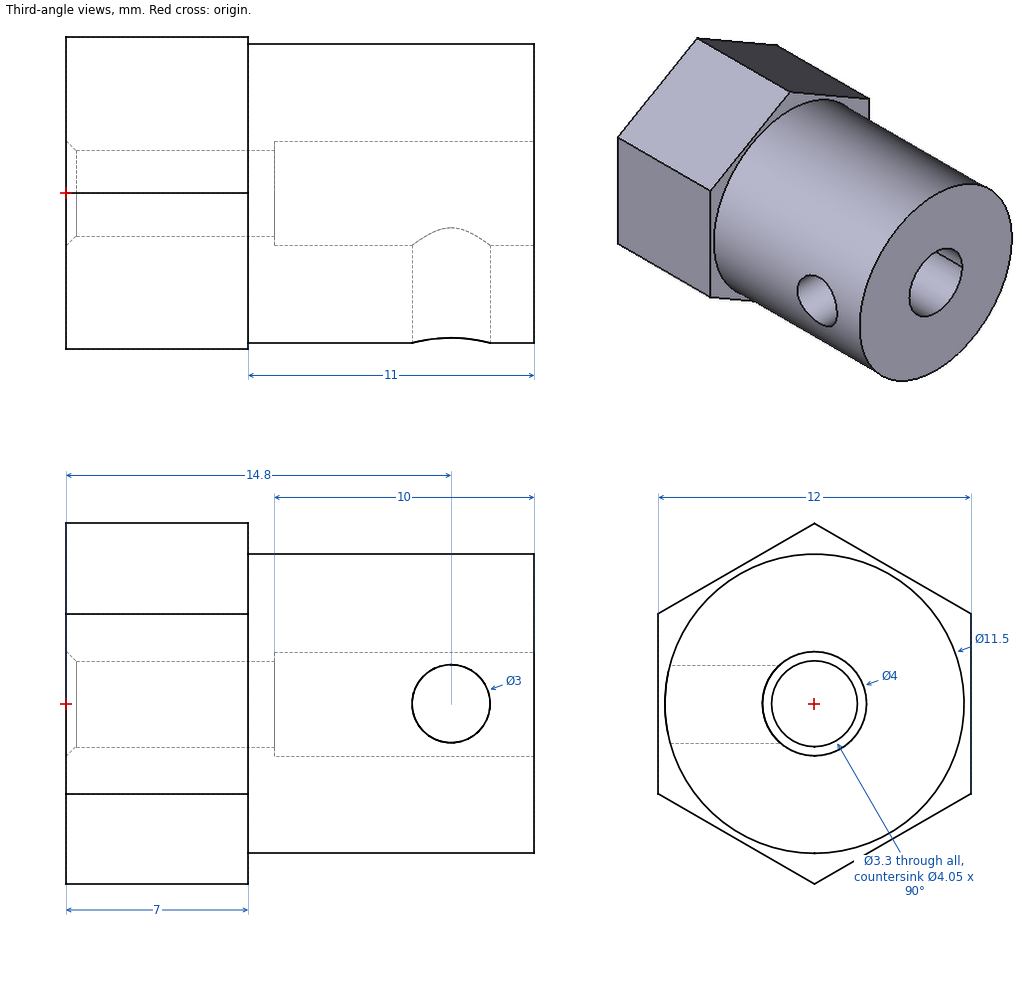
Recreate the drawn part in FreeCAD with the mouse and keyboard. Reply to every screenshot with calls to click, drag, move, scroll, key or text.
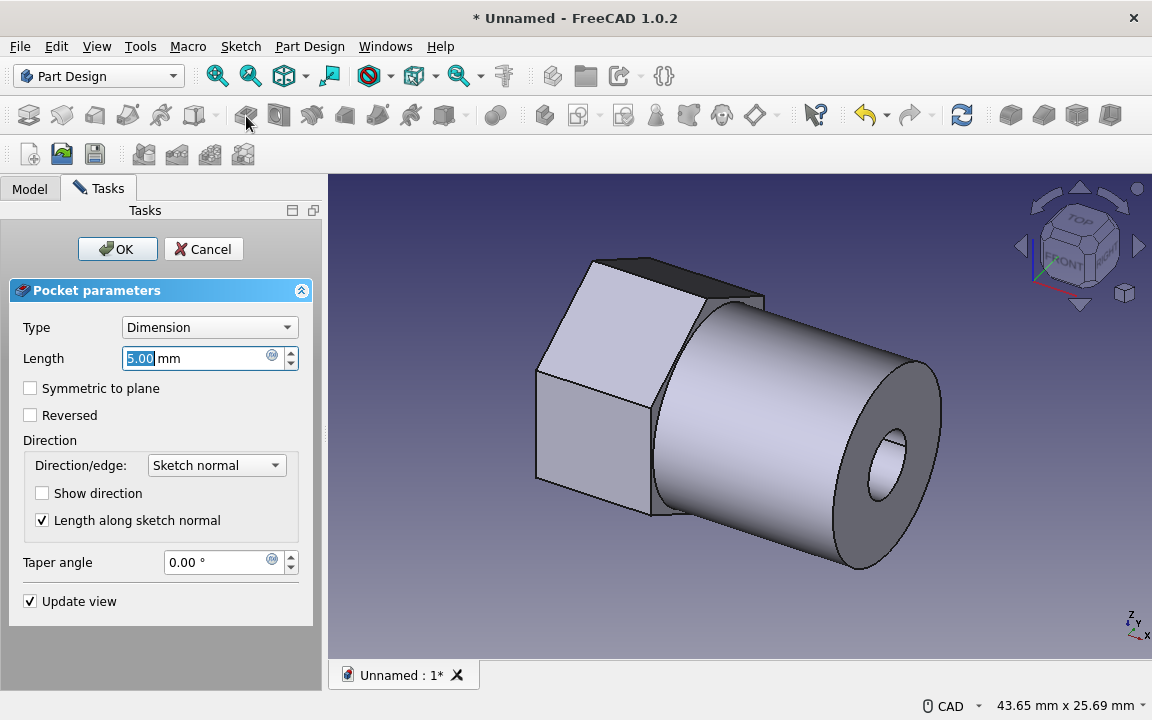
click(210, 328)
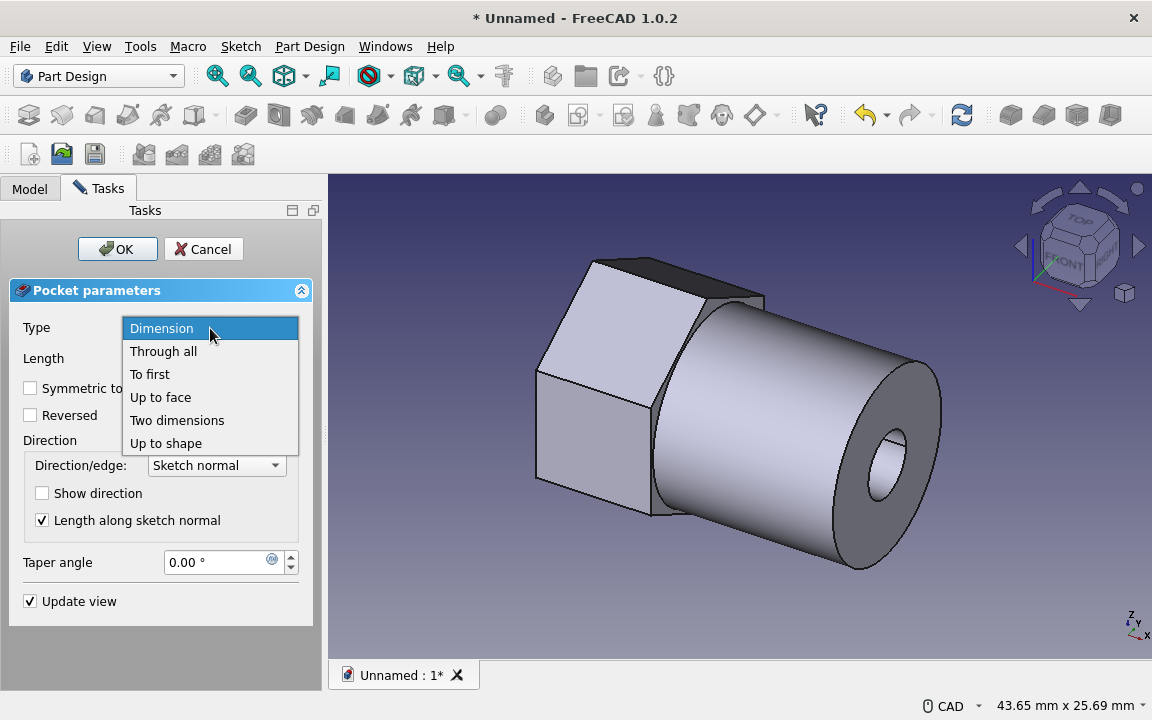
click(208, 352)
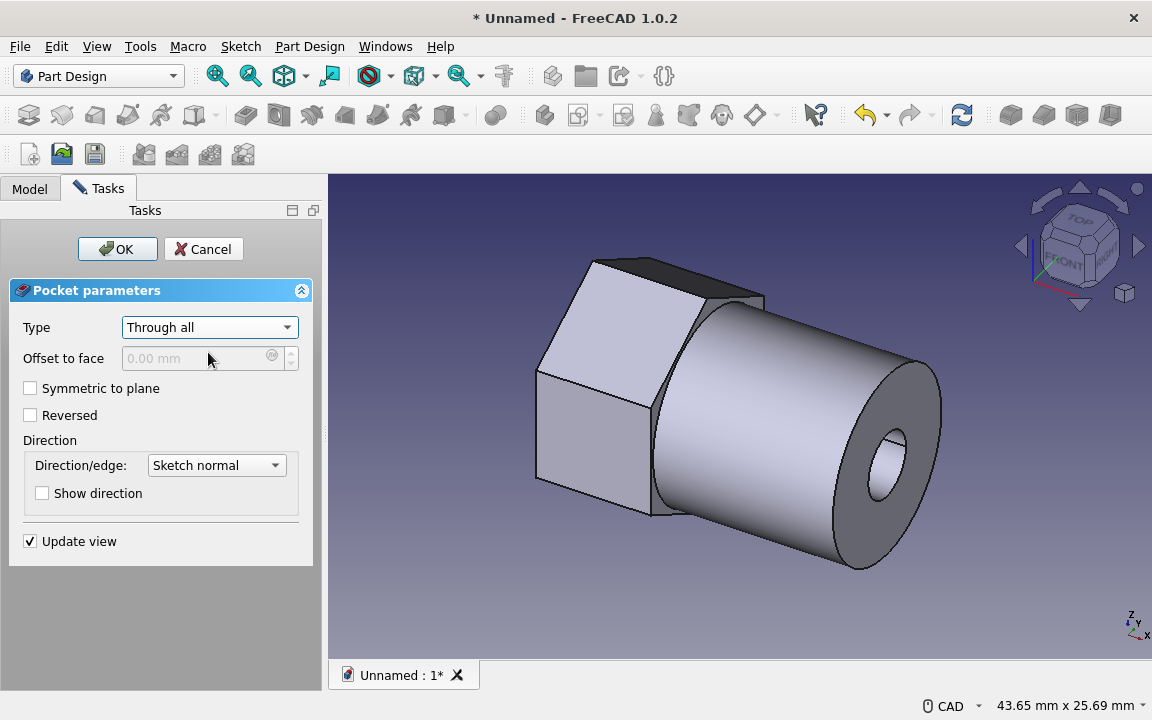
click(31, 415)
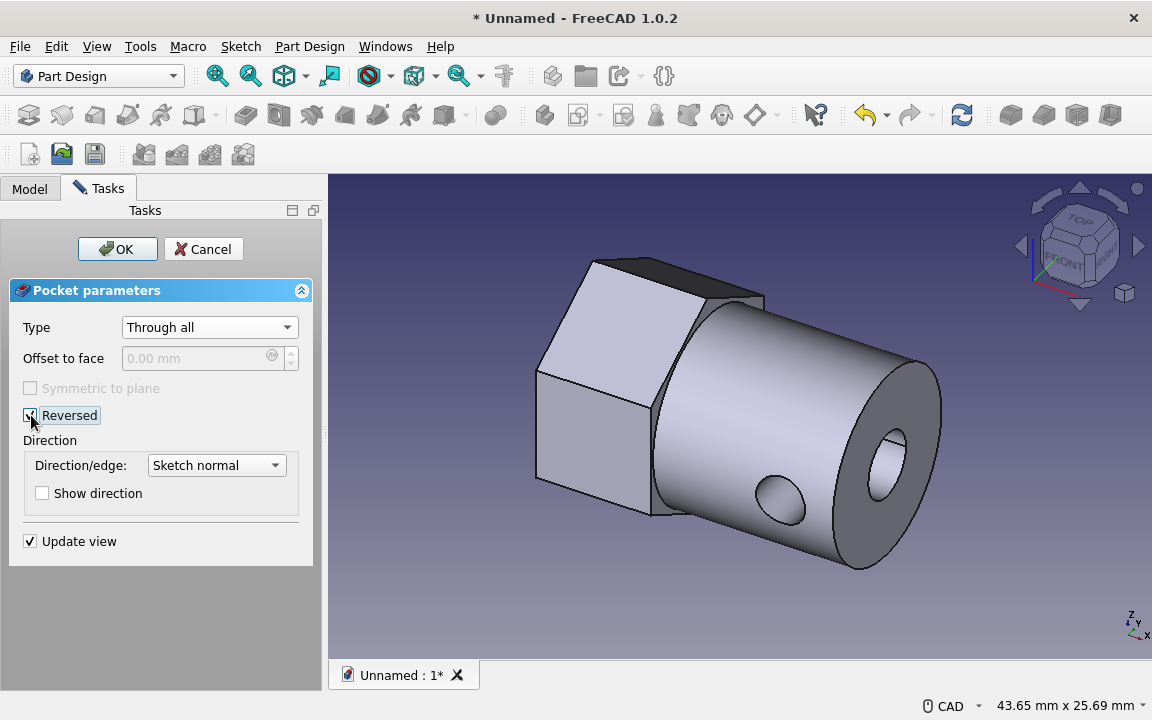
click(118, 249)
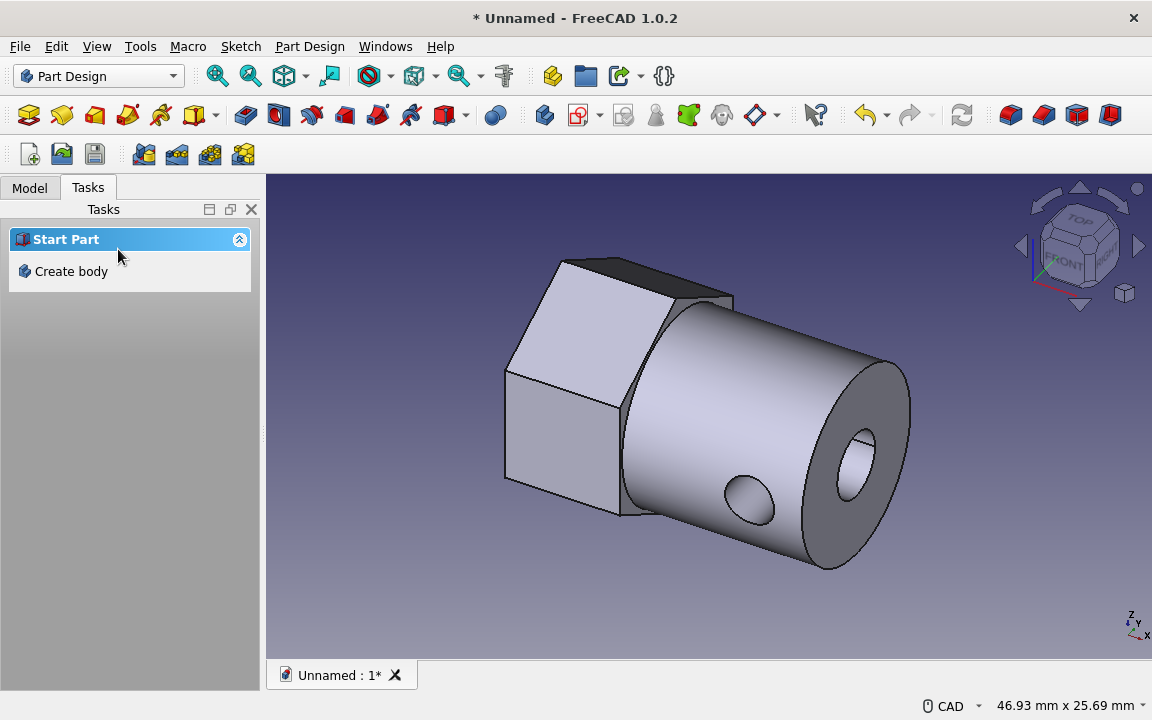
key(0)